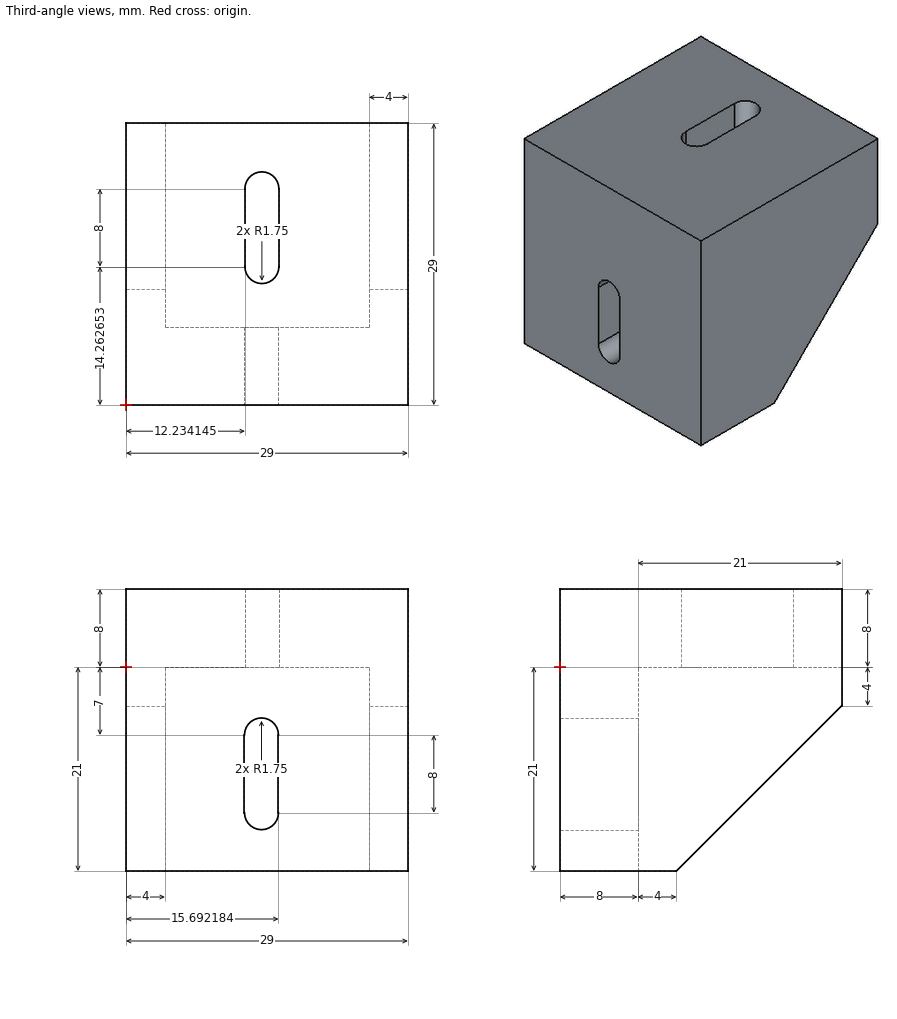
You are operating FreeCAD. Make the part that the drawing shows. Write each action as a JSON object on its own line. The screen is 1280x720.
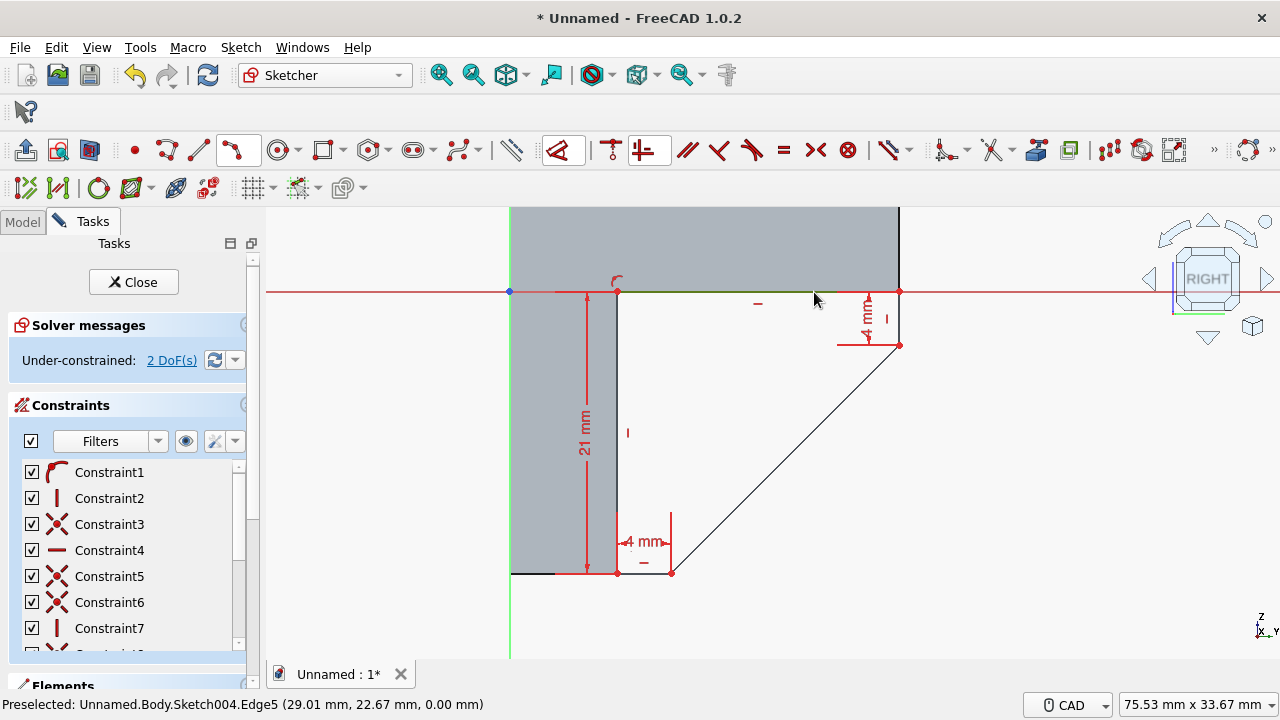
{"action": "left_click", "coordinate": [580, 150]}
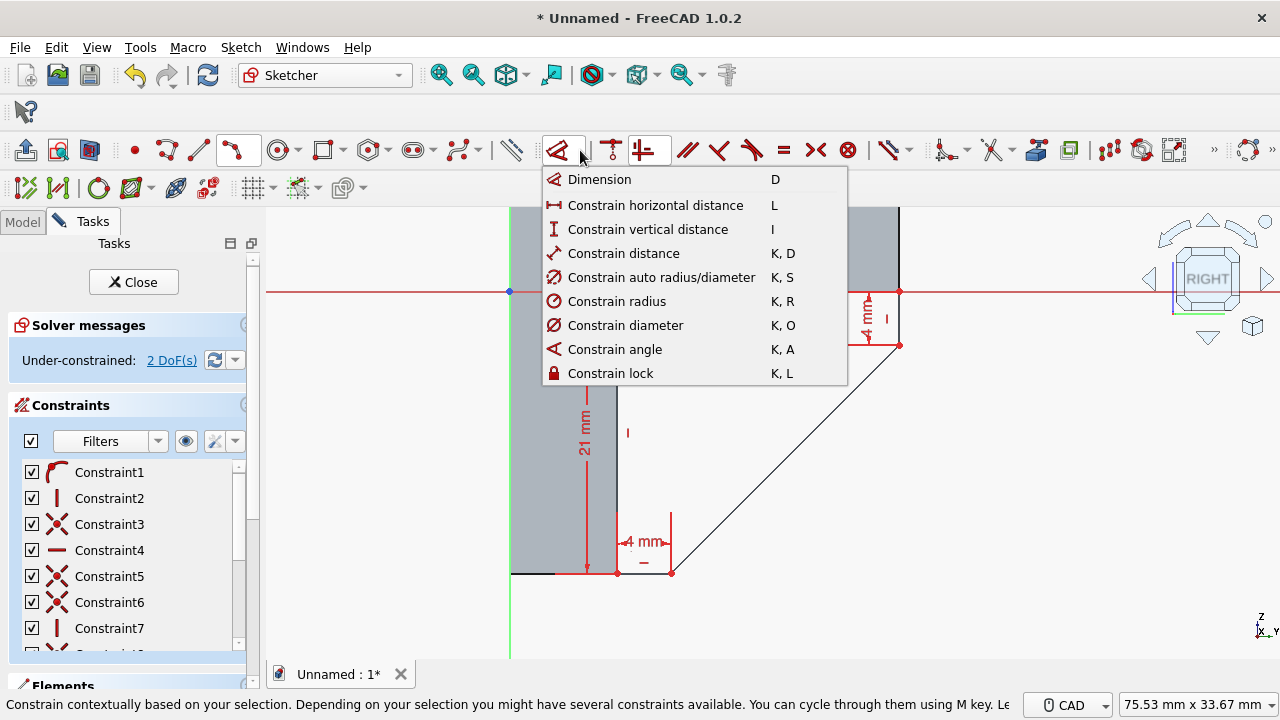
{"action": "left_click", "coordinate": [695, 205]}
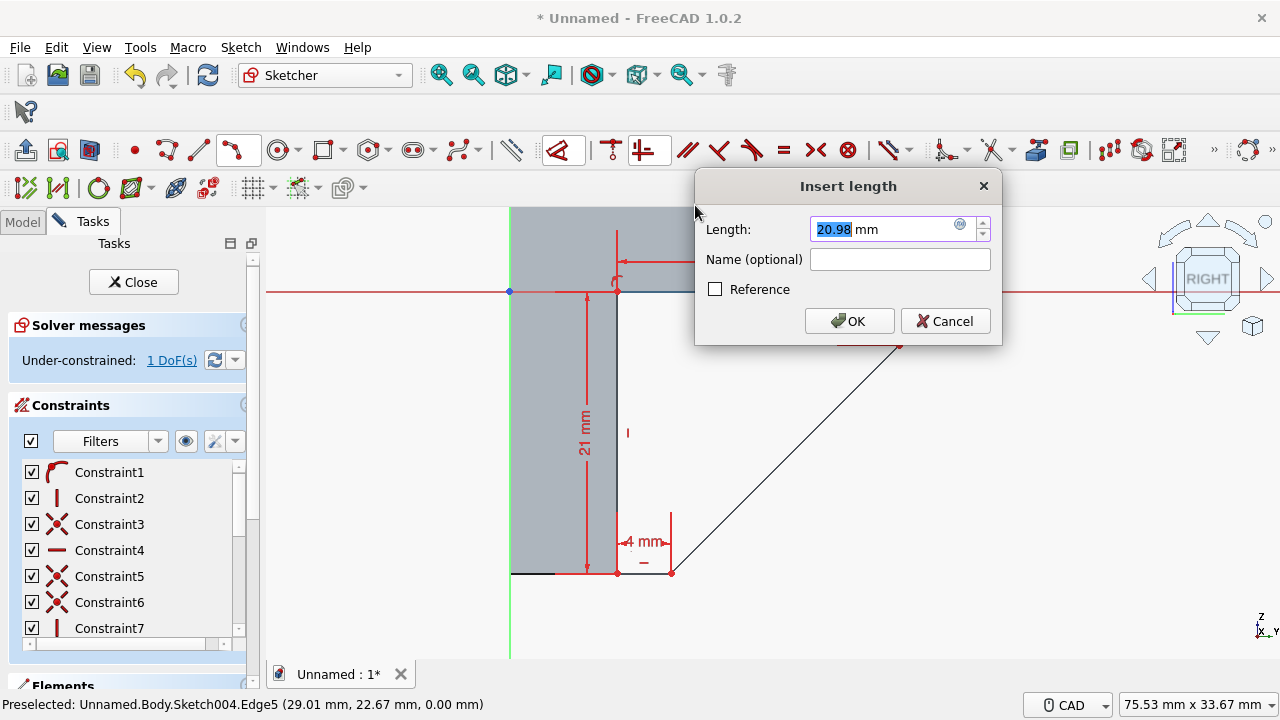
{"action": "type", "text": "21"}
{"action": "key", "text": "Return"}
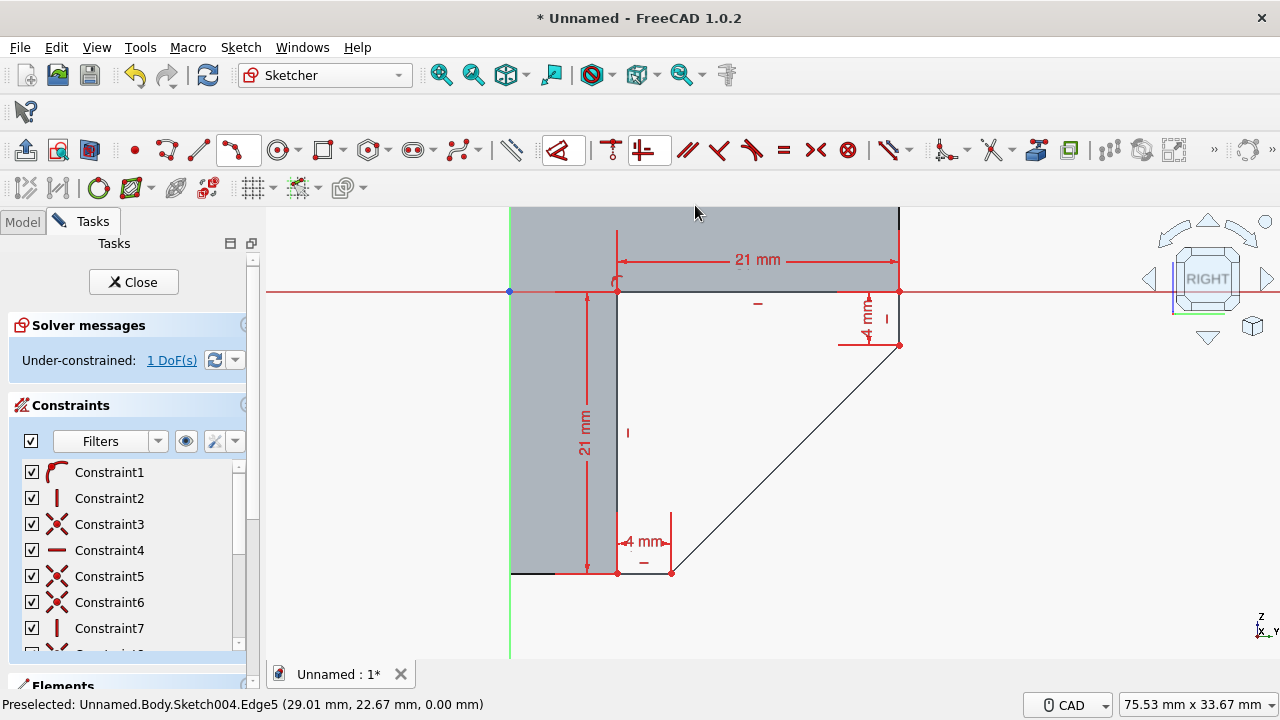
{"action": "left_click", "coordinate": [617, 292]}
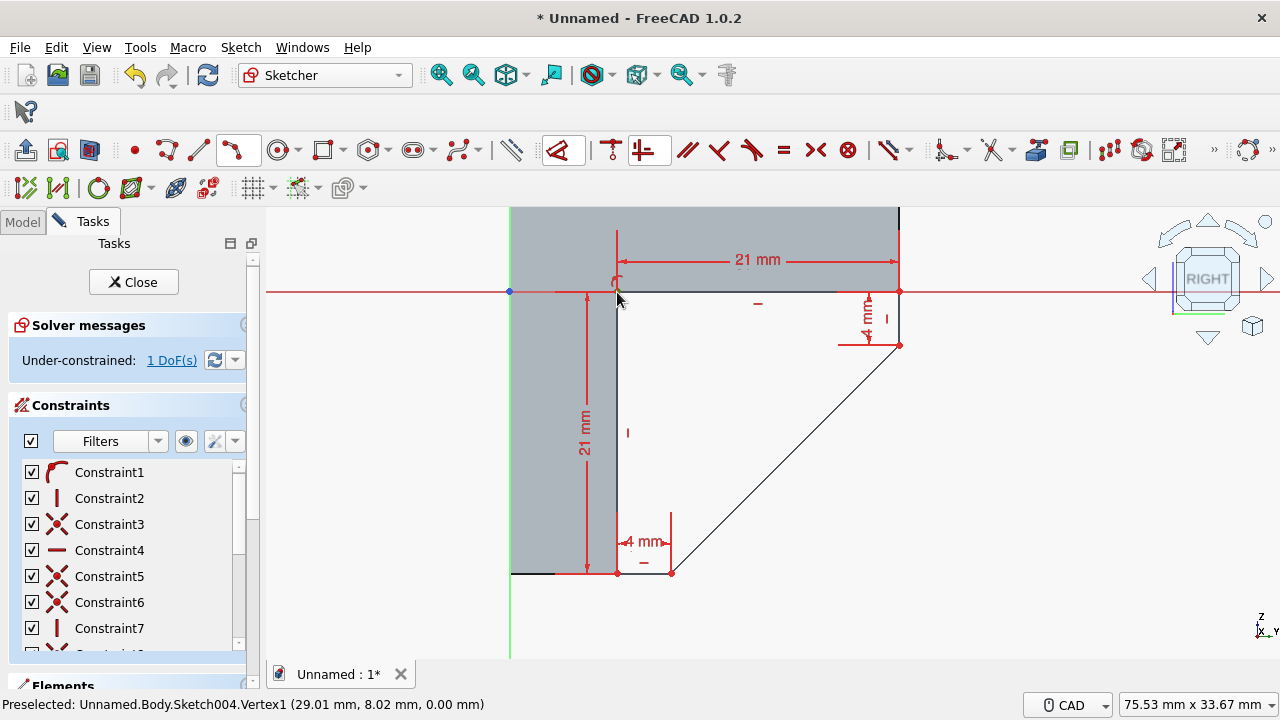
{"action": "left_click", "coordinate": [580, 150]}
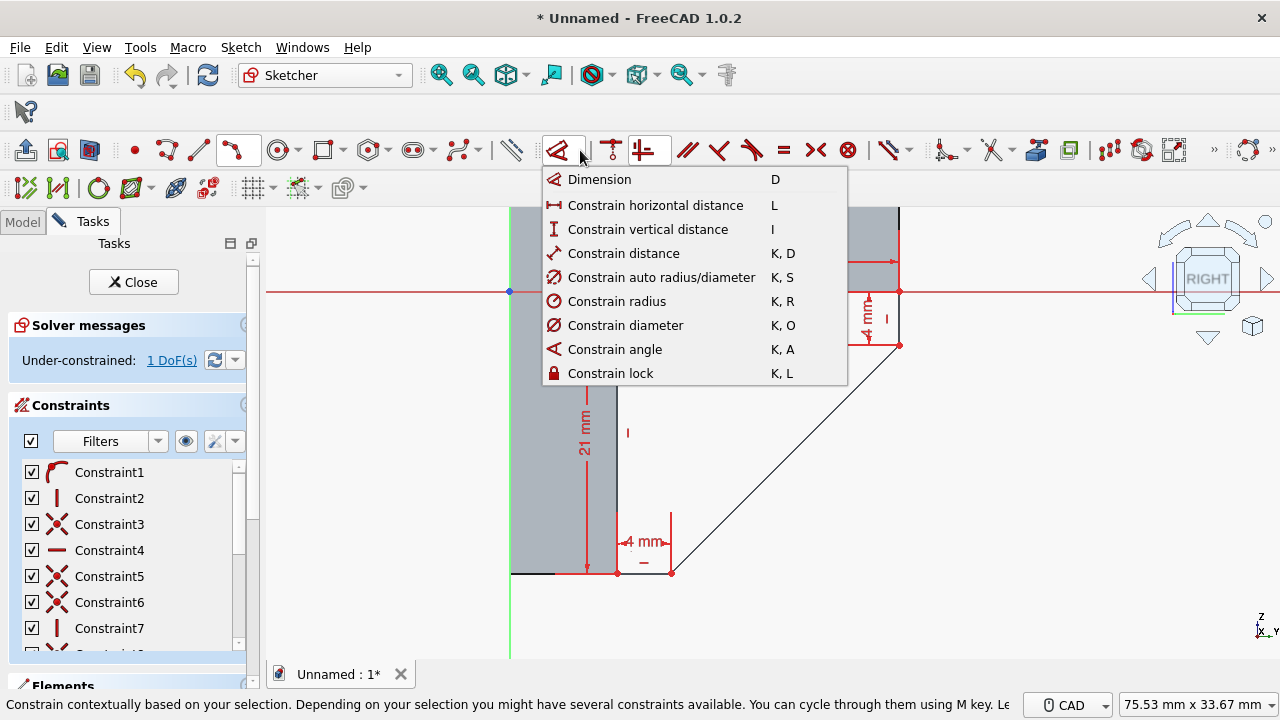
{"action": "left_click", "coordinate": [695, 205]}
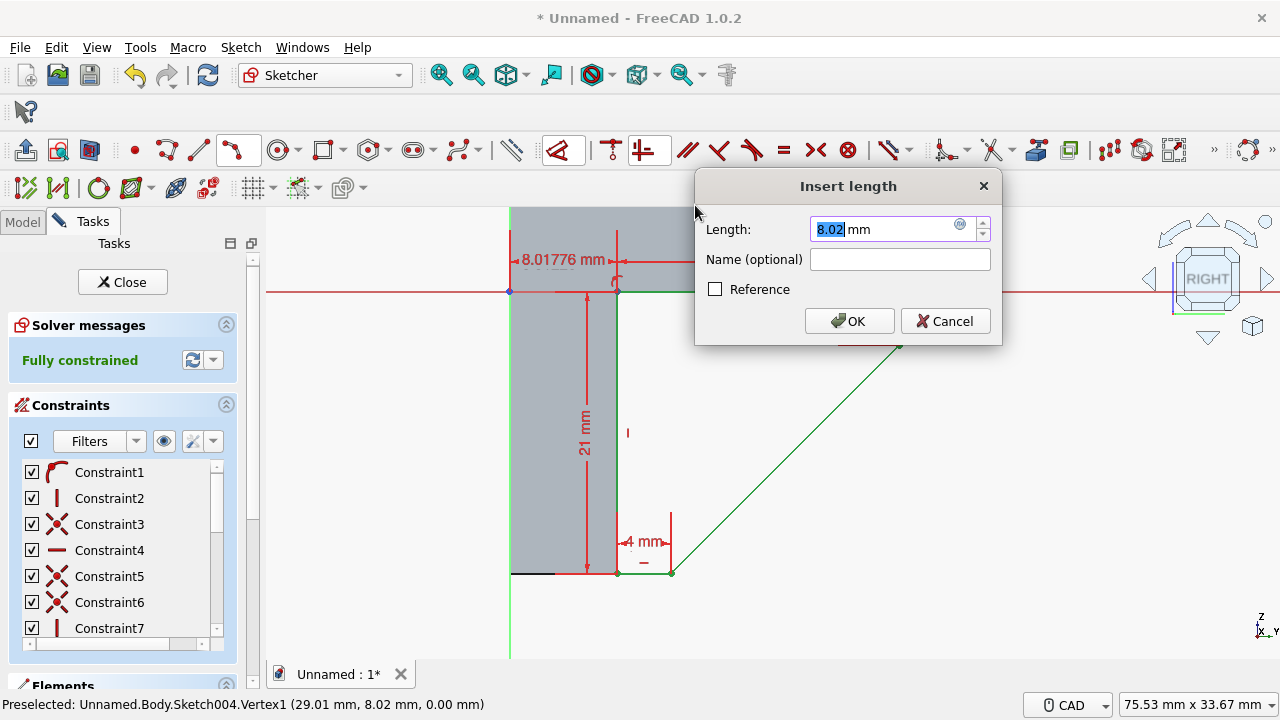
{"action": "type", "text": "8"}
{"action": "key", "text": "Return"}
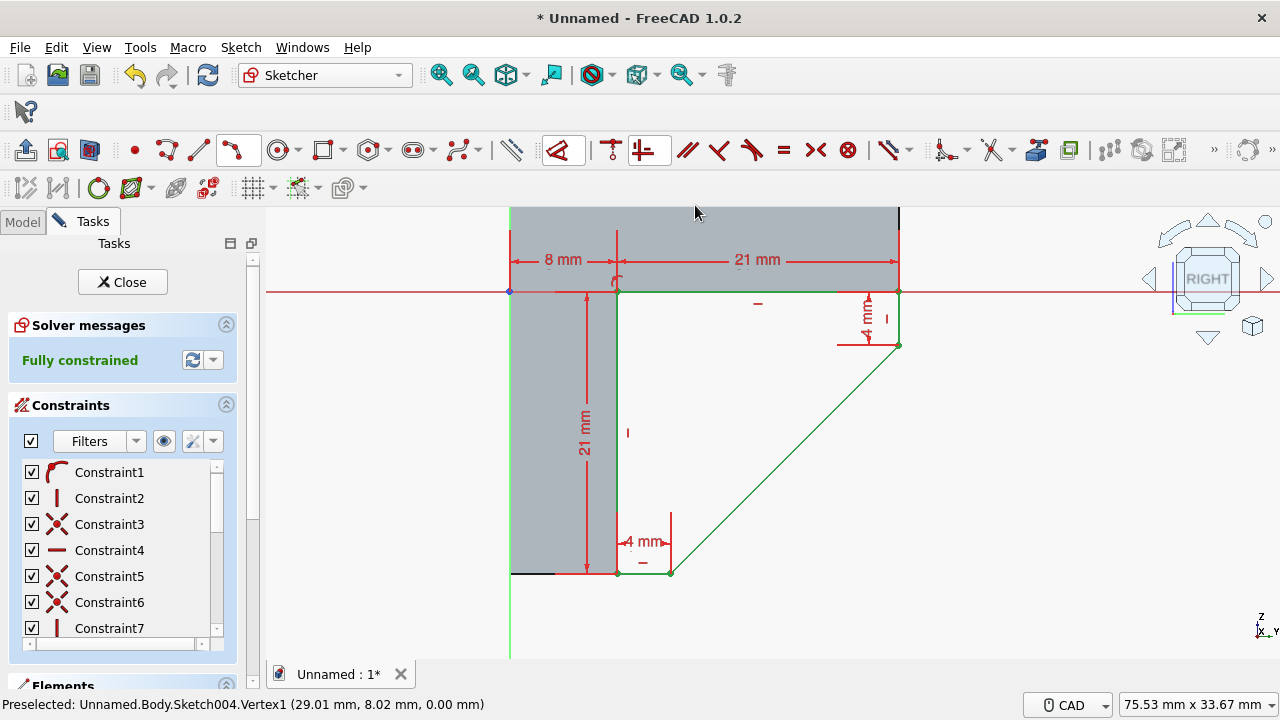
{"action": "left_click", "coordinate": [123, 282]}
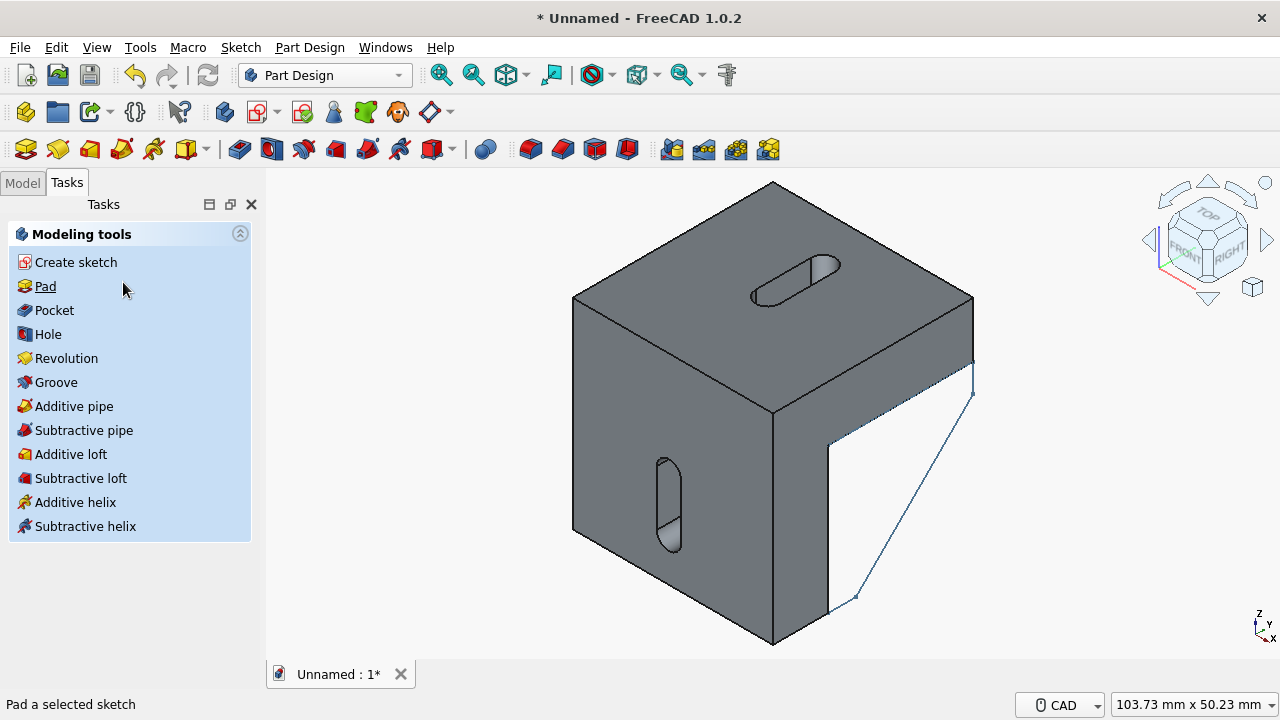
{"action": "left_click", "coordinate": [26, 150]}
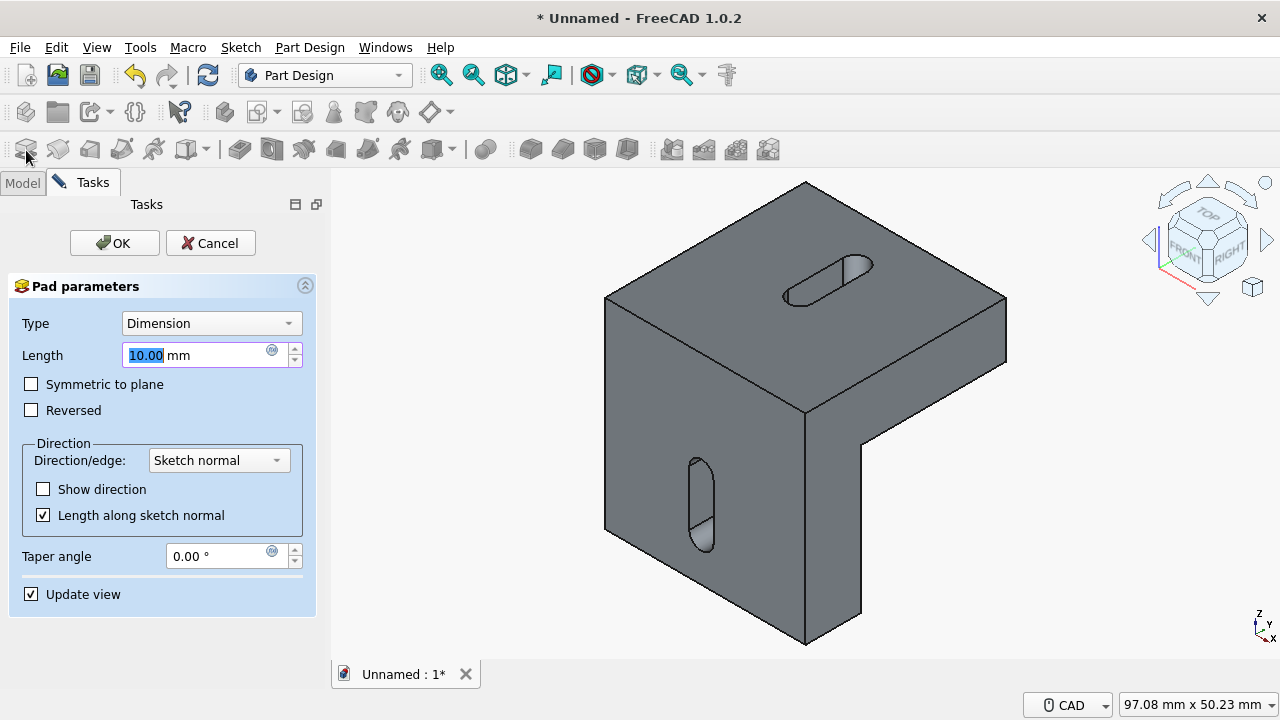
{"action": "type", "text": "4"}
{"action": "key", "text": "Tab"}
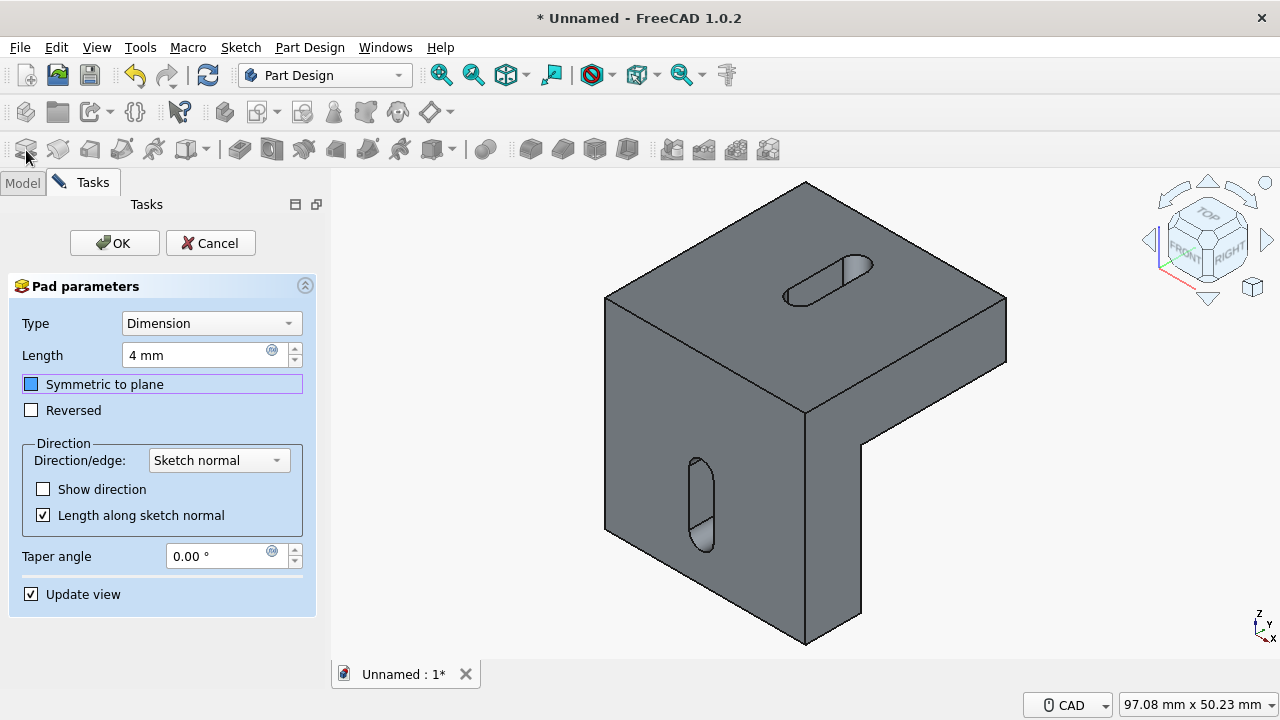
{"action": "left_click", "coordinate": [30, 410]}